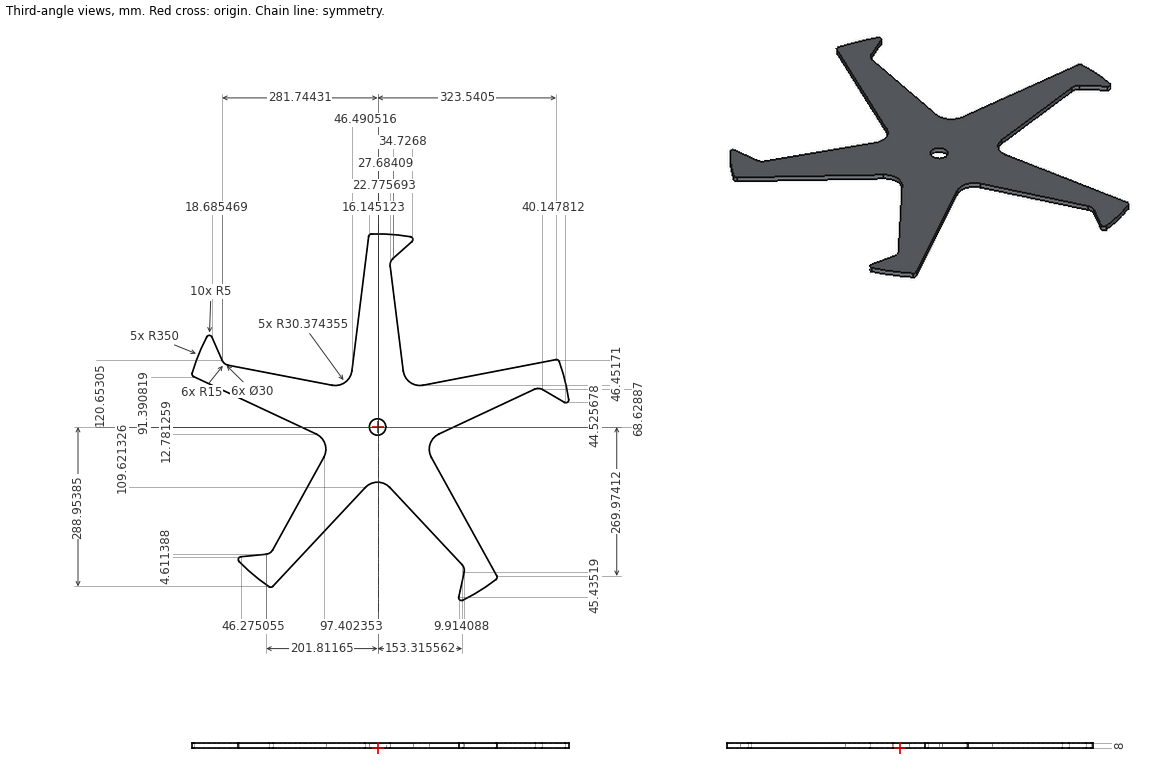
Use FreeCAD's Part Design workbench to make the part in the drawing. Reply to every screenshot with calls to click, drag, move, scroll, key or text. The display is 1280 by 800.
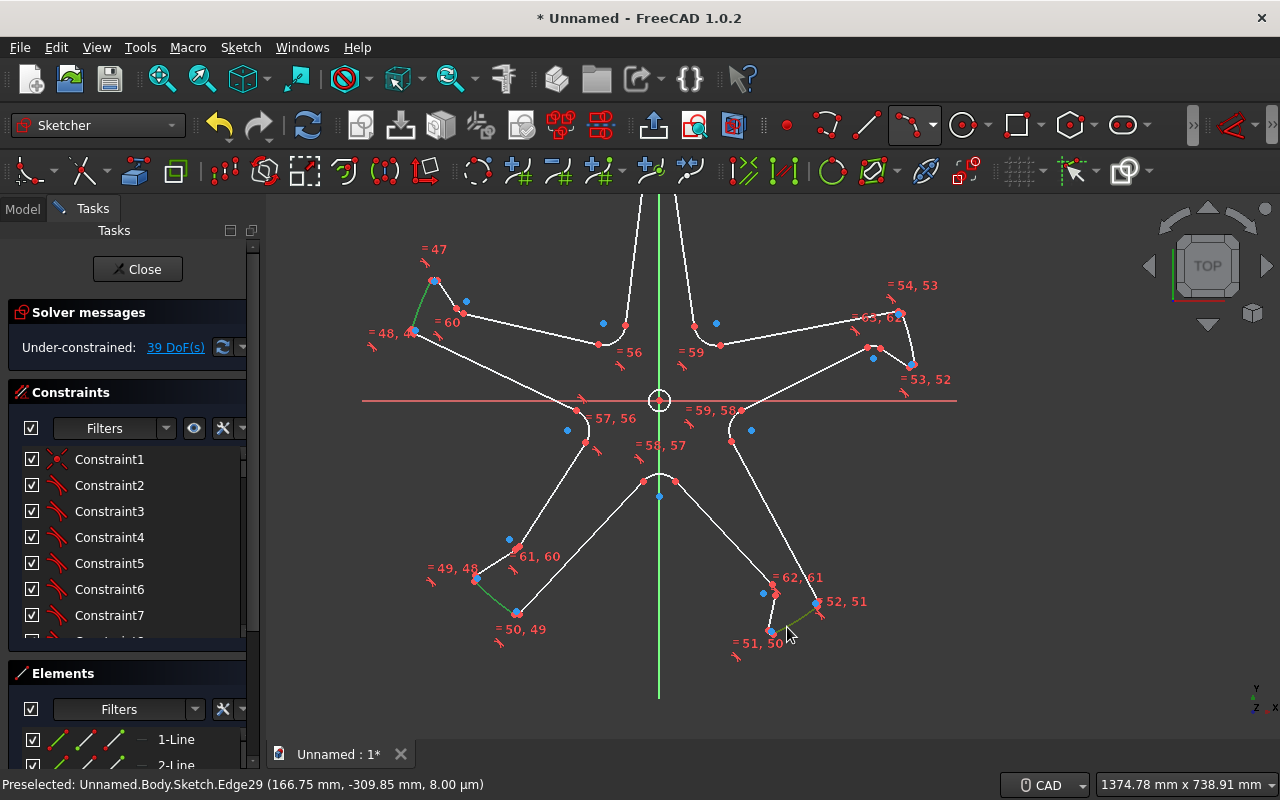
click(912, 349)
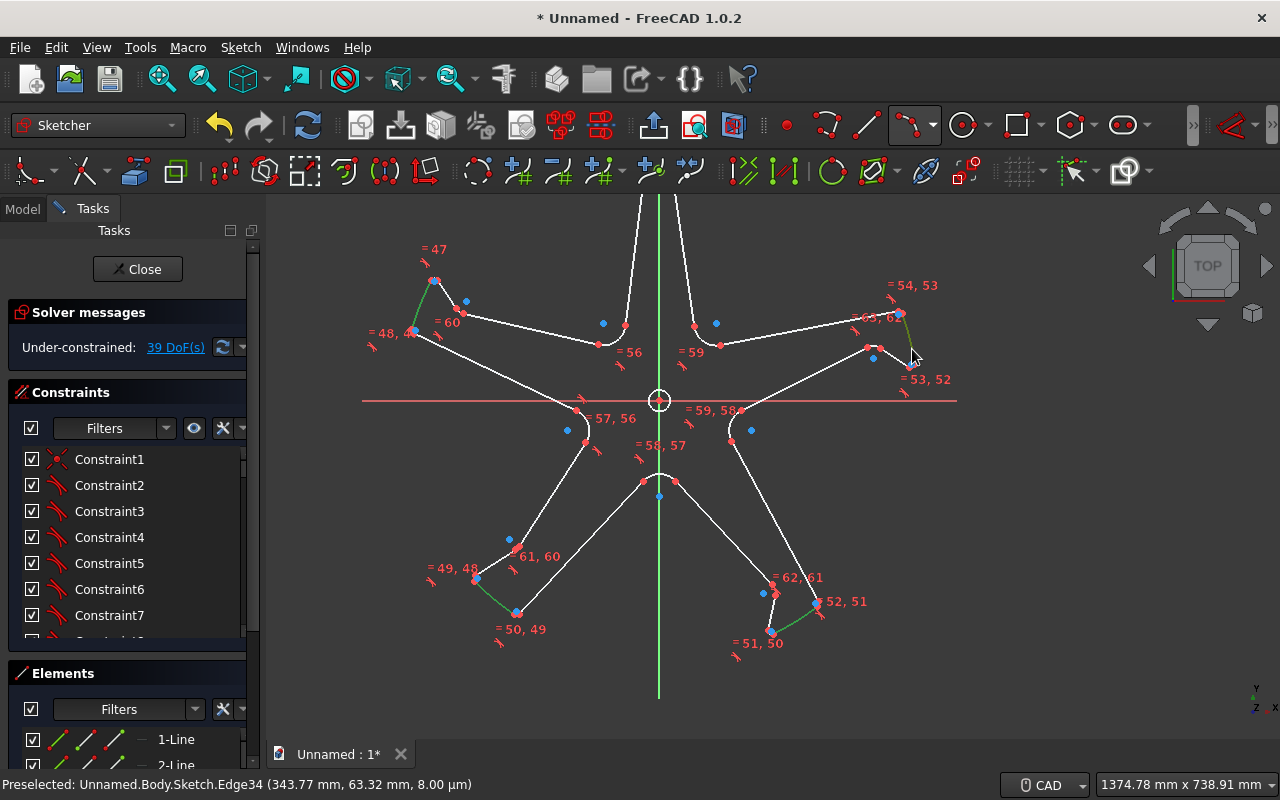
scroll(788, 627, down, 2)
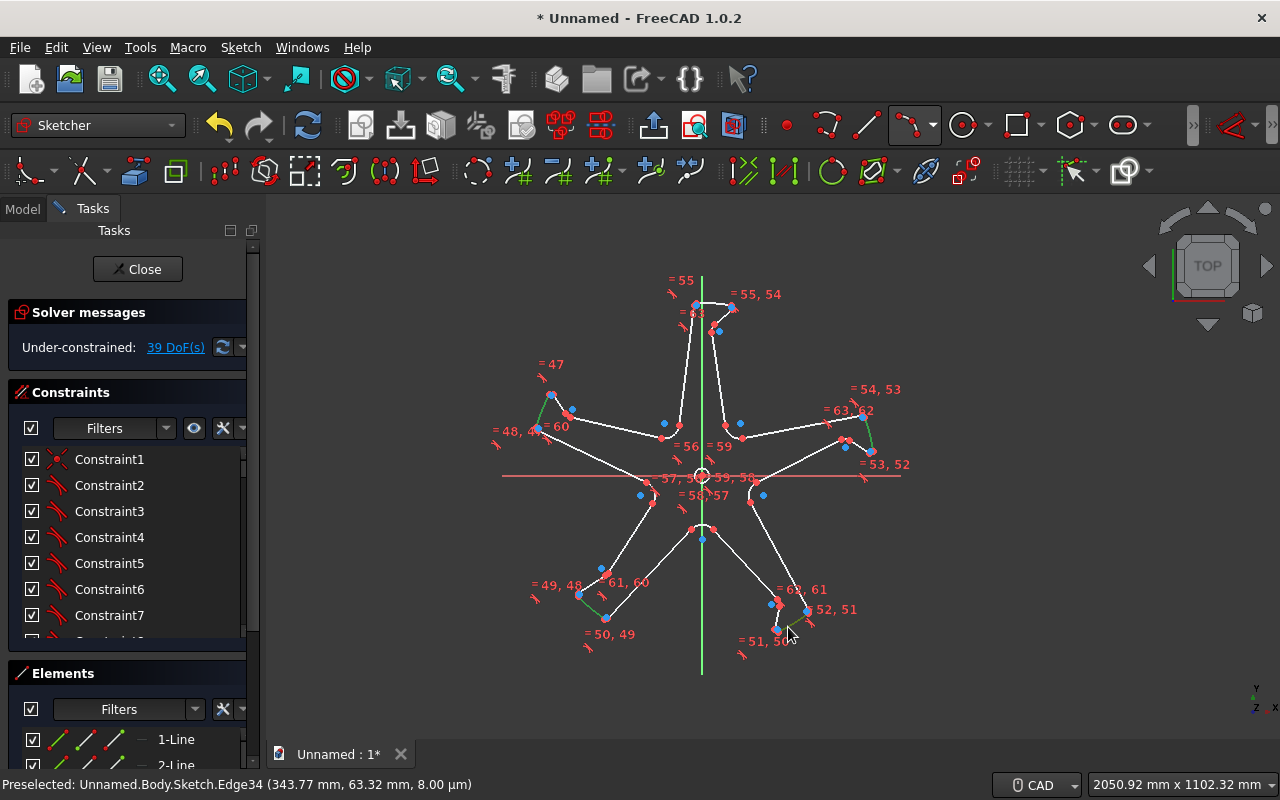
scroll(721, 304, up, 2)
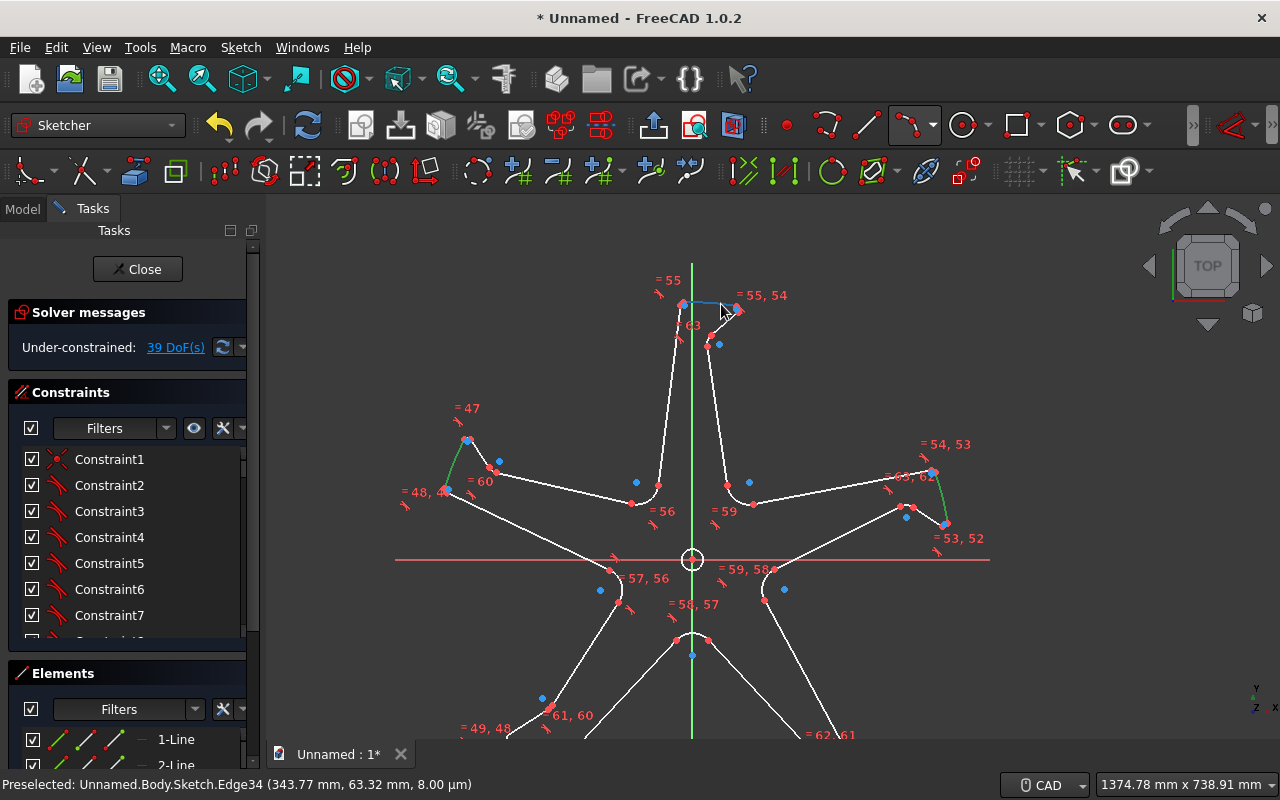
click(721, 304)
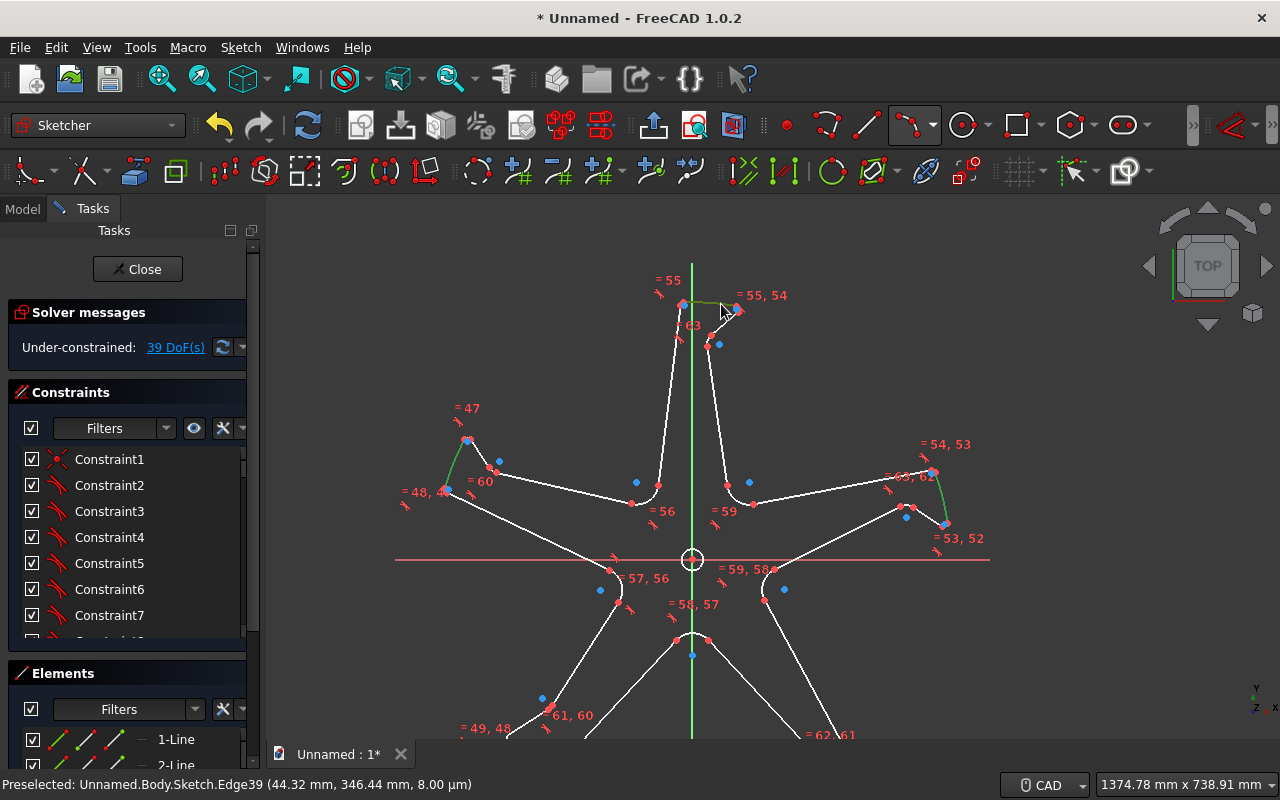
key(e)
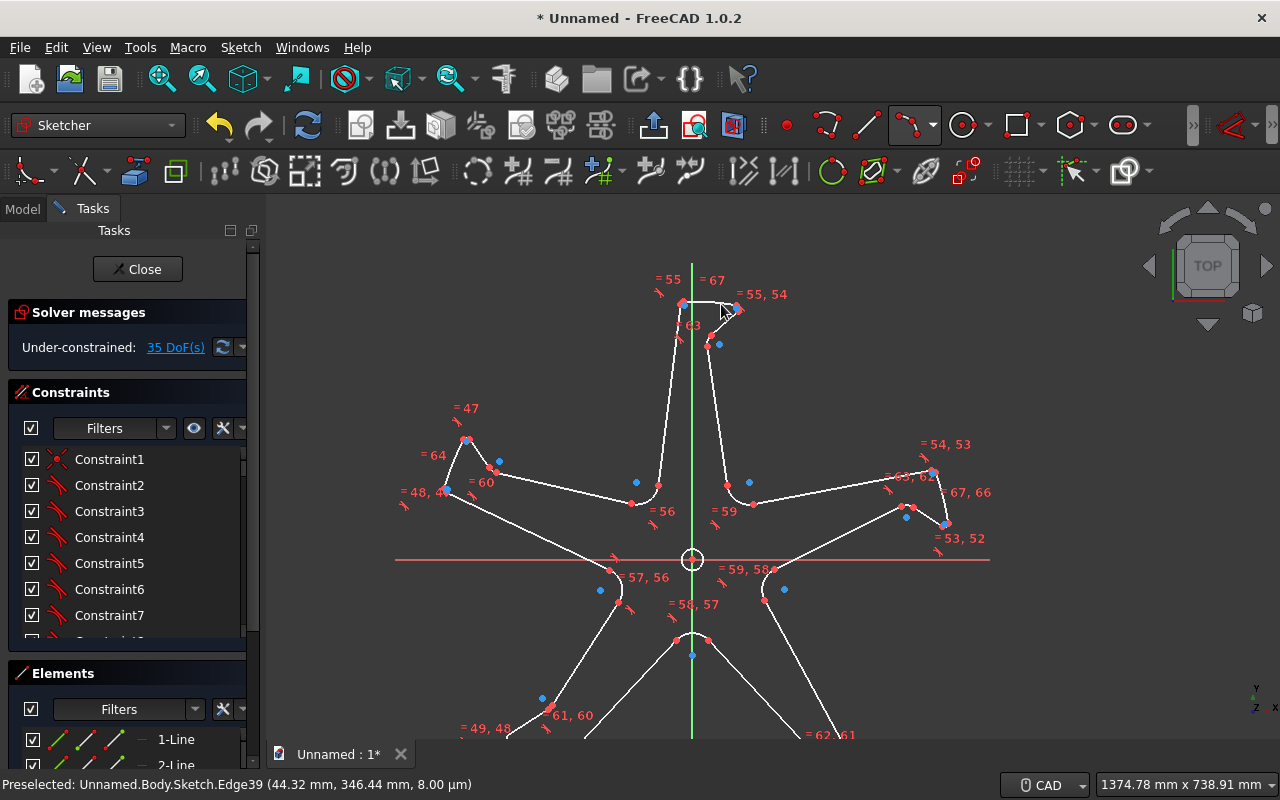
click(693, 655)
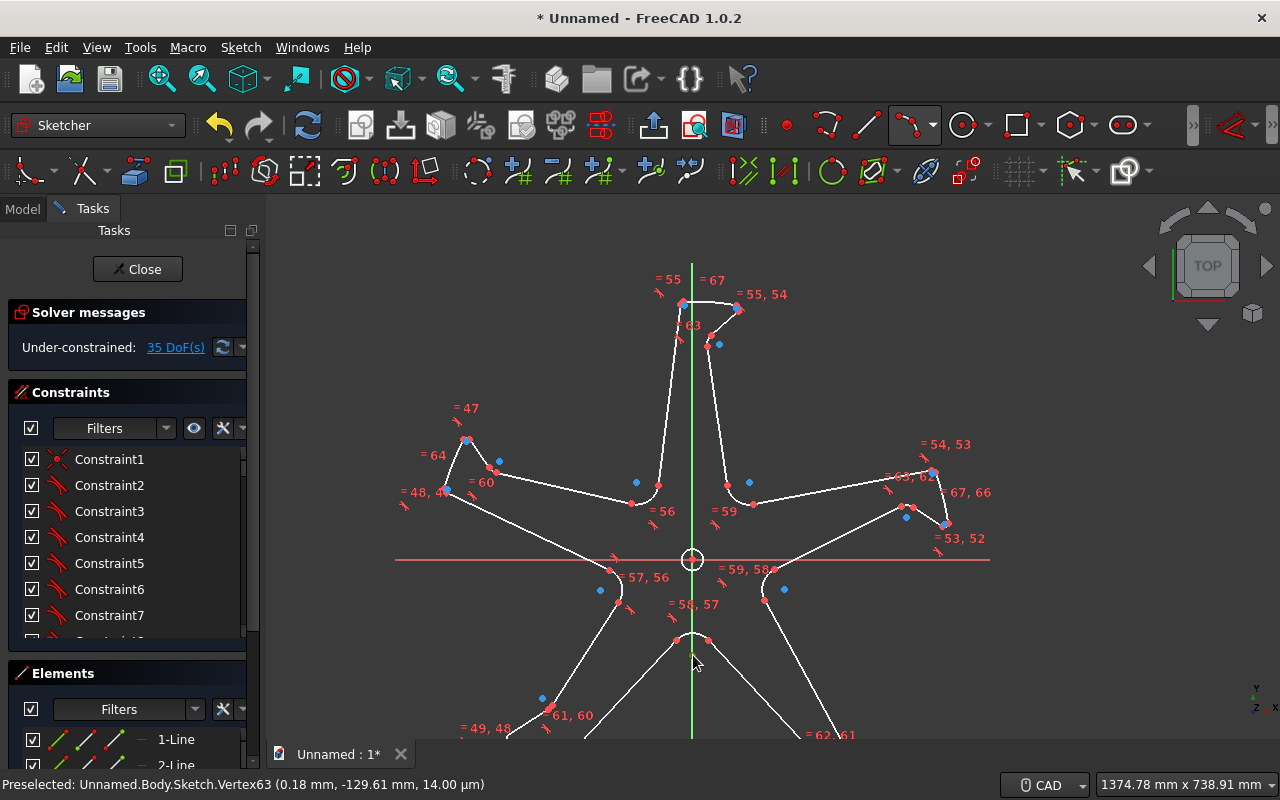
click(692, 676)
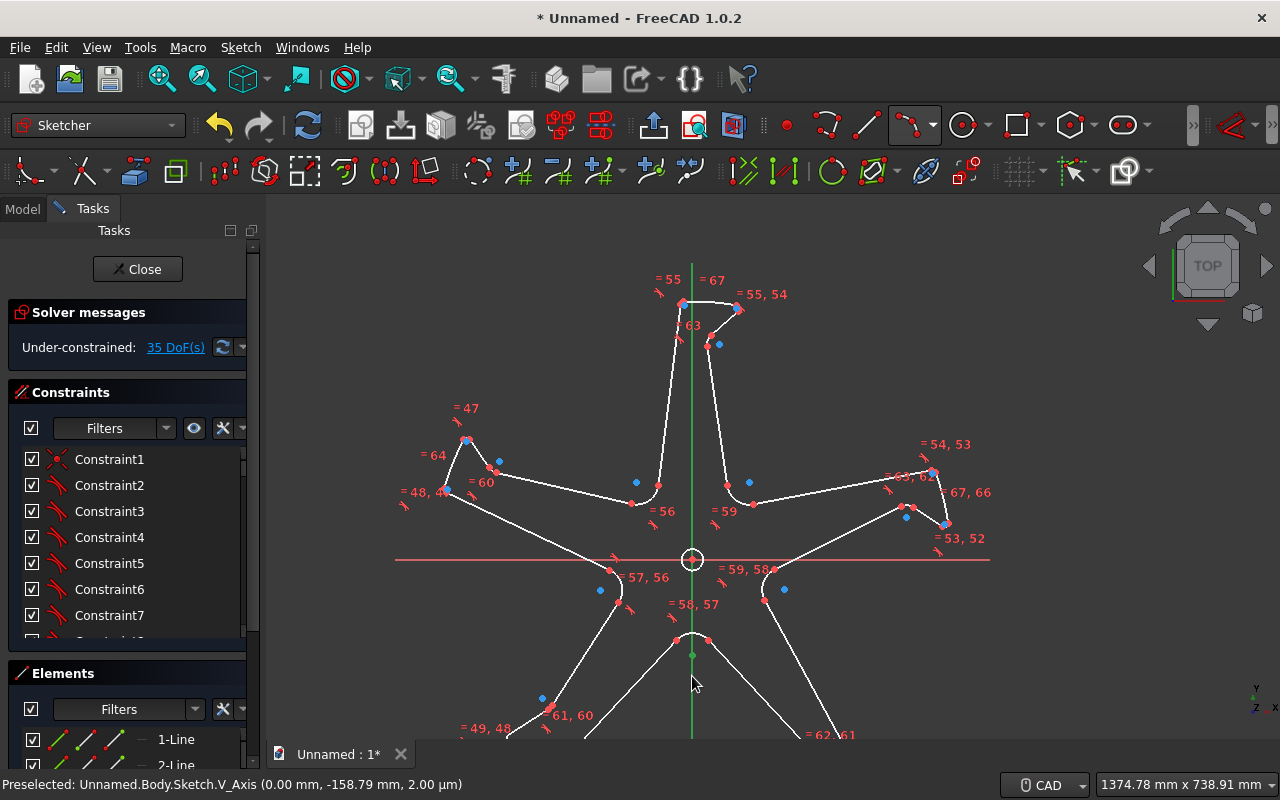
key(c)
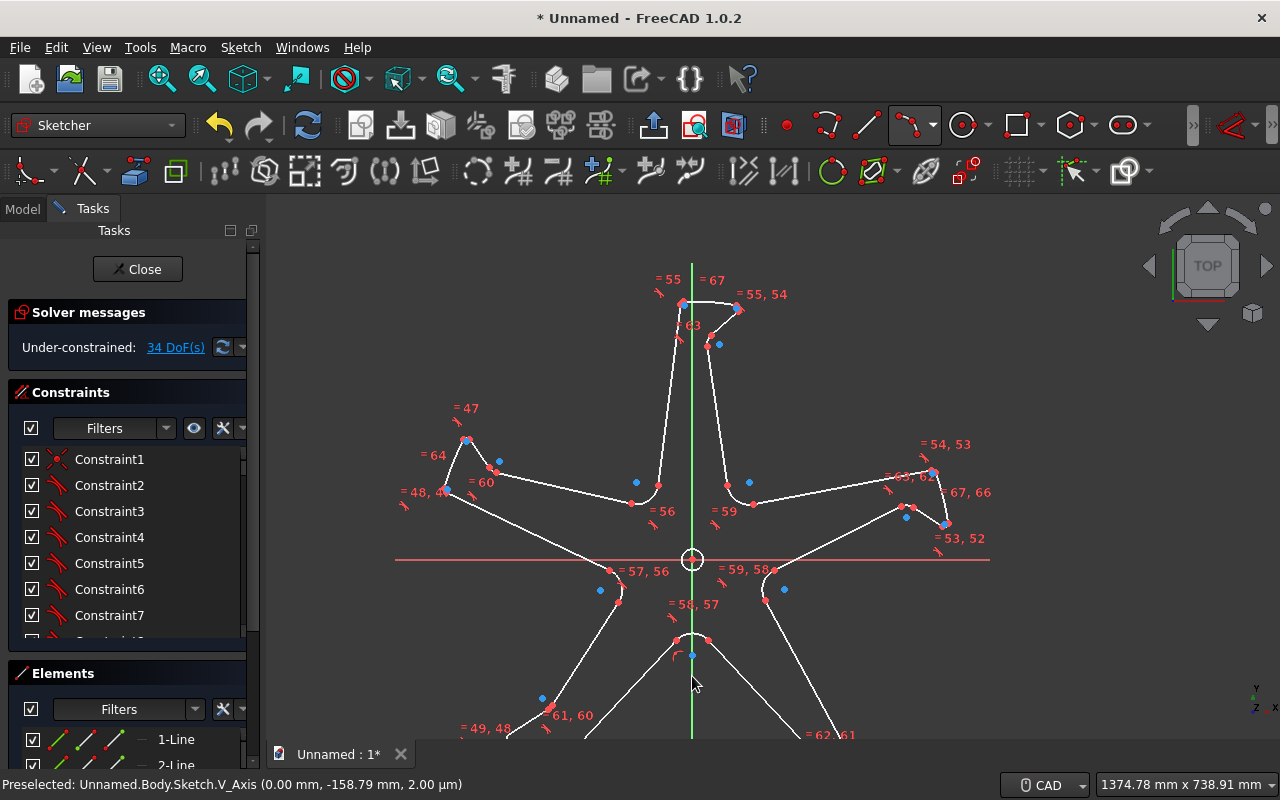
click(600, 590)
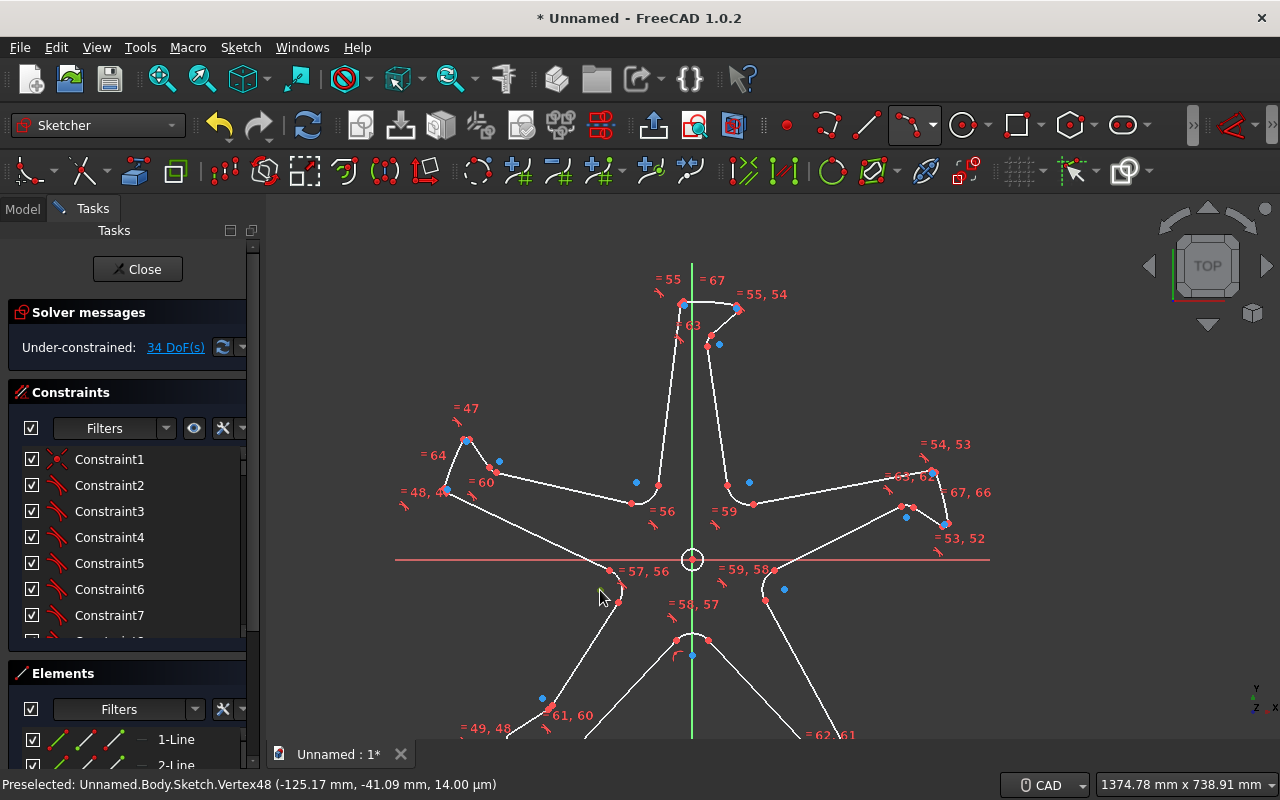
click(784, 590)